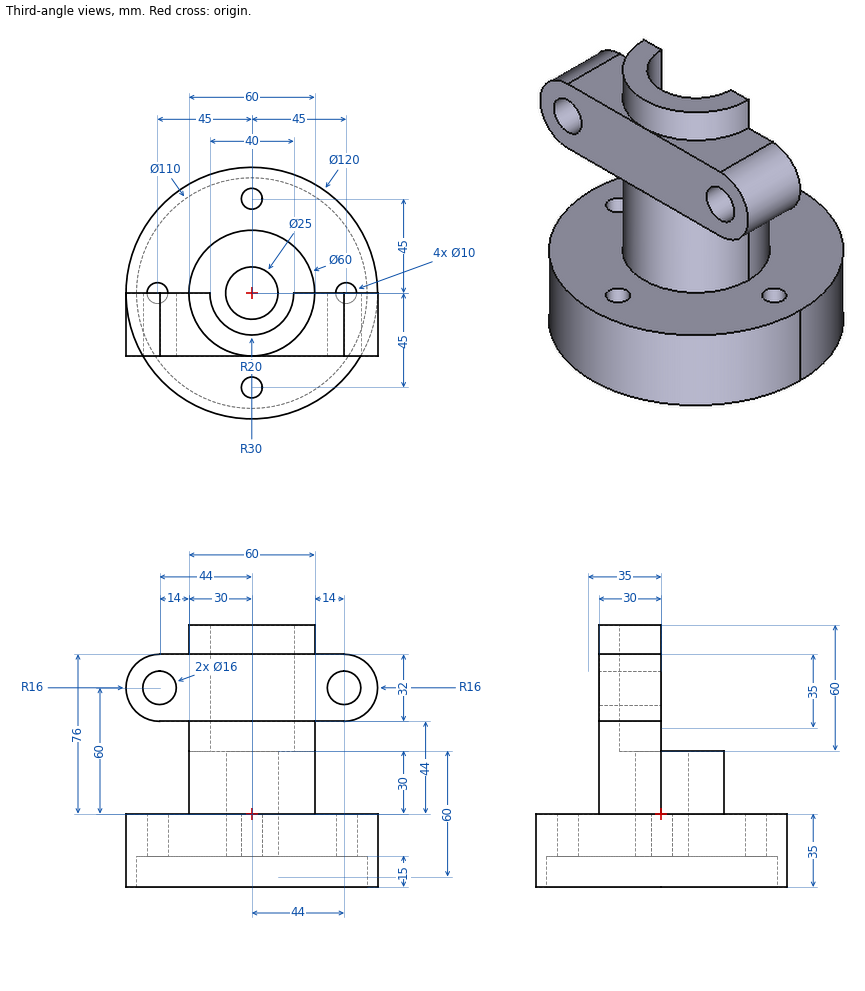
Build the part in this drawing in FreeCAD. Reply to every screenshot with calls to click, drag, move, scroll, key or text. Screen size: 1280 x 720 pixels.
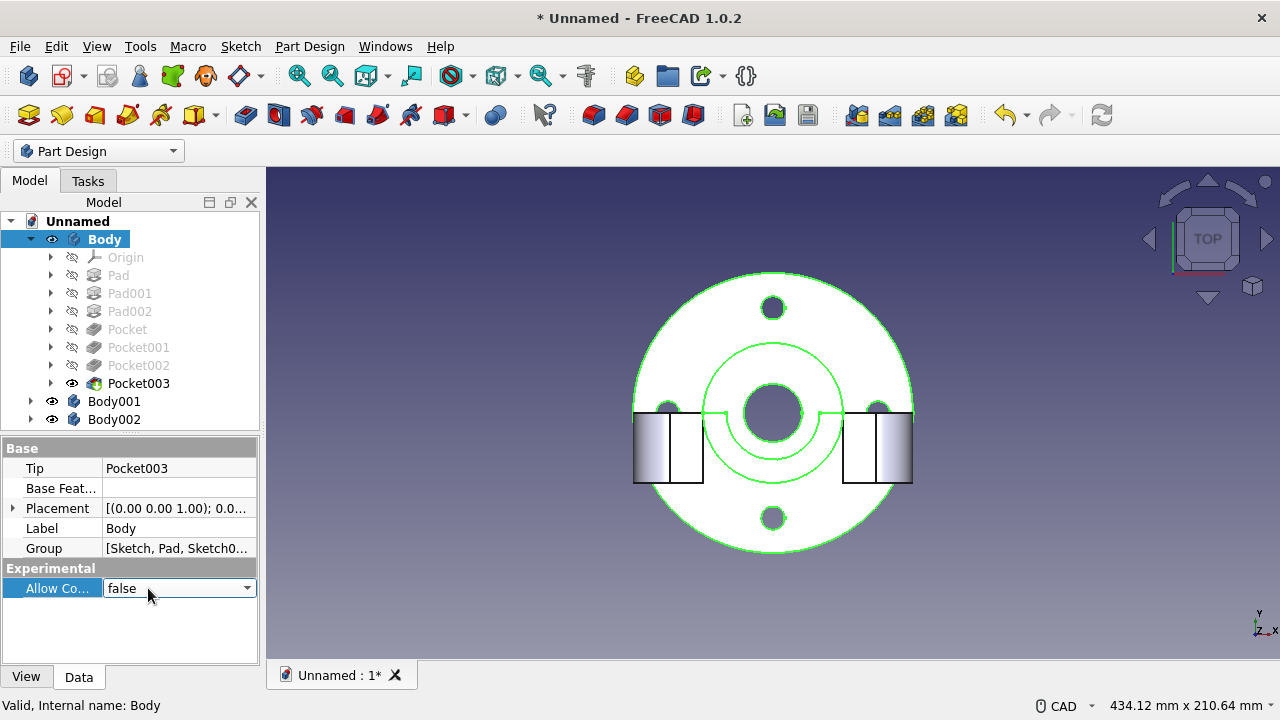
click(148, 588)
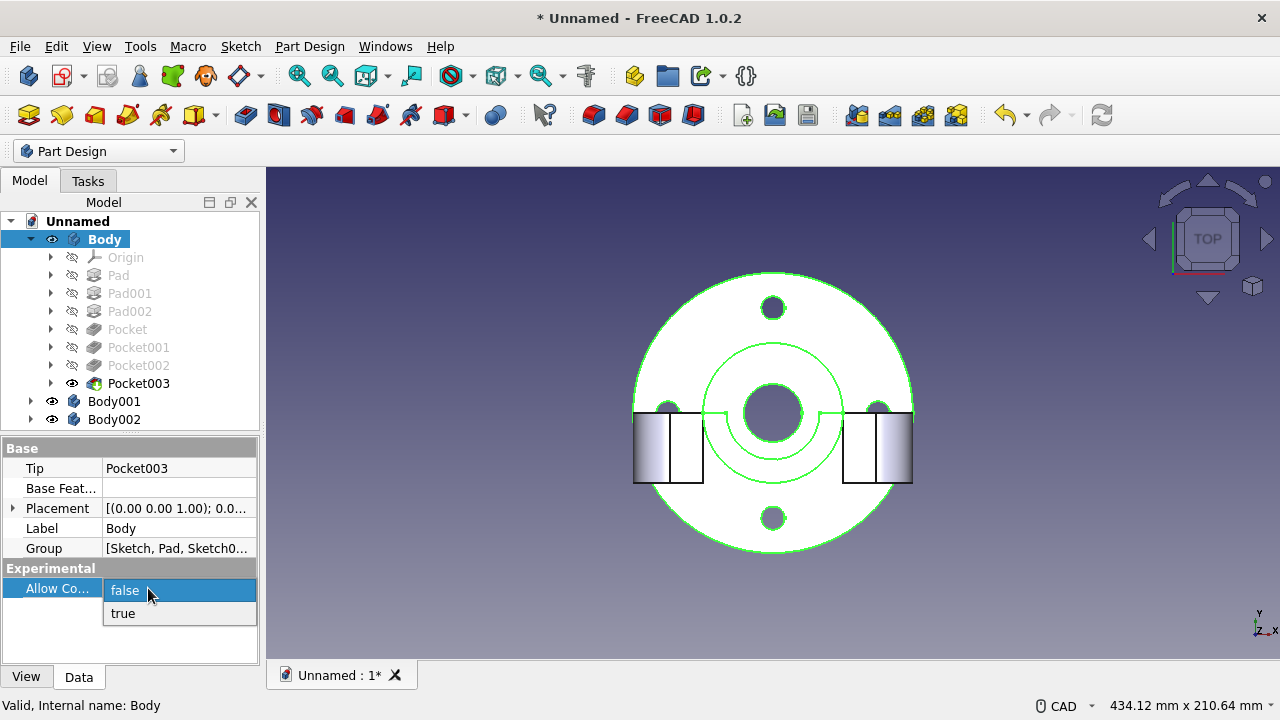
click(178, 614)
key(Return)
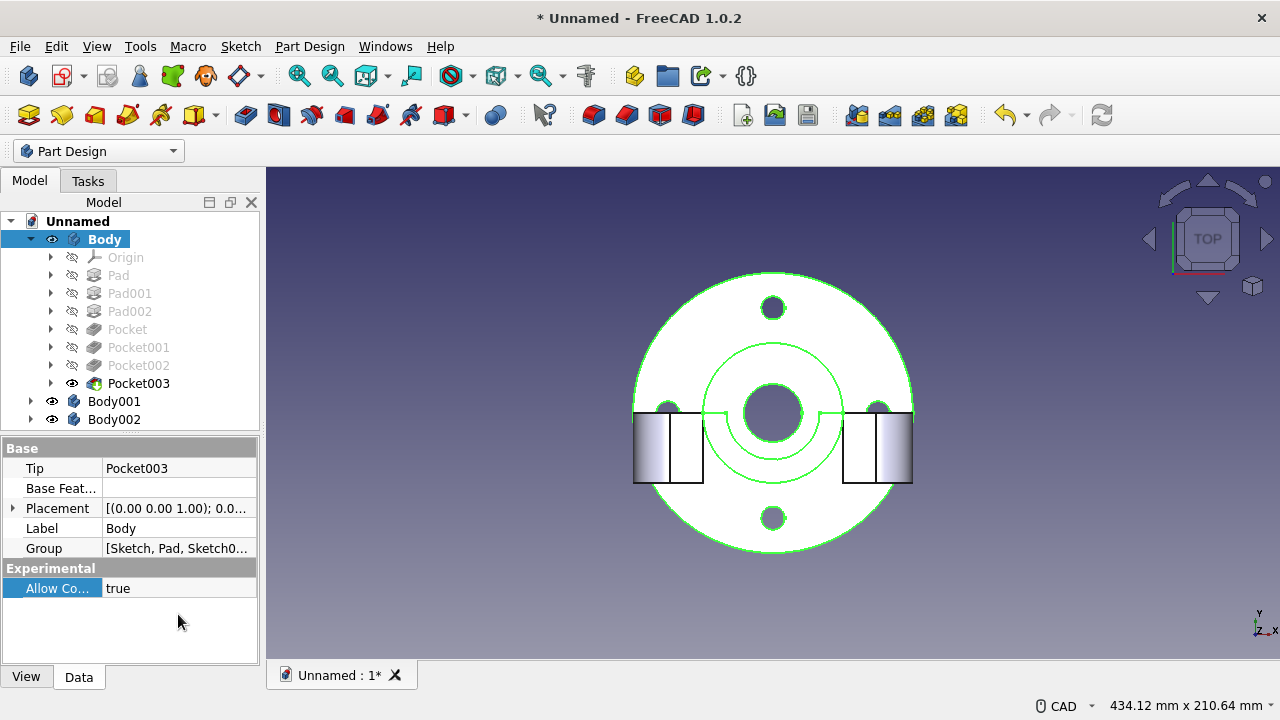
click(97, 401)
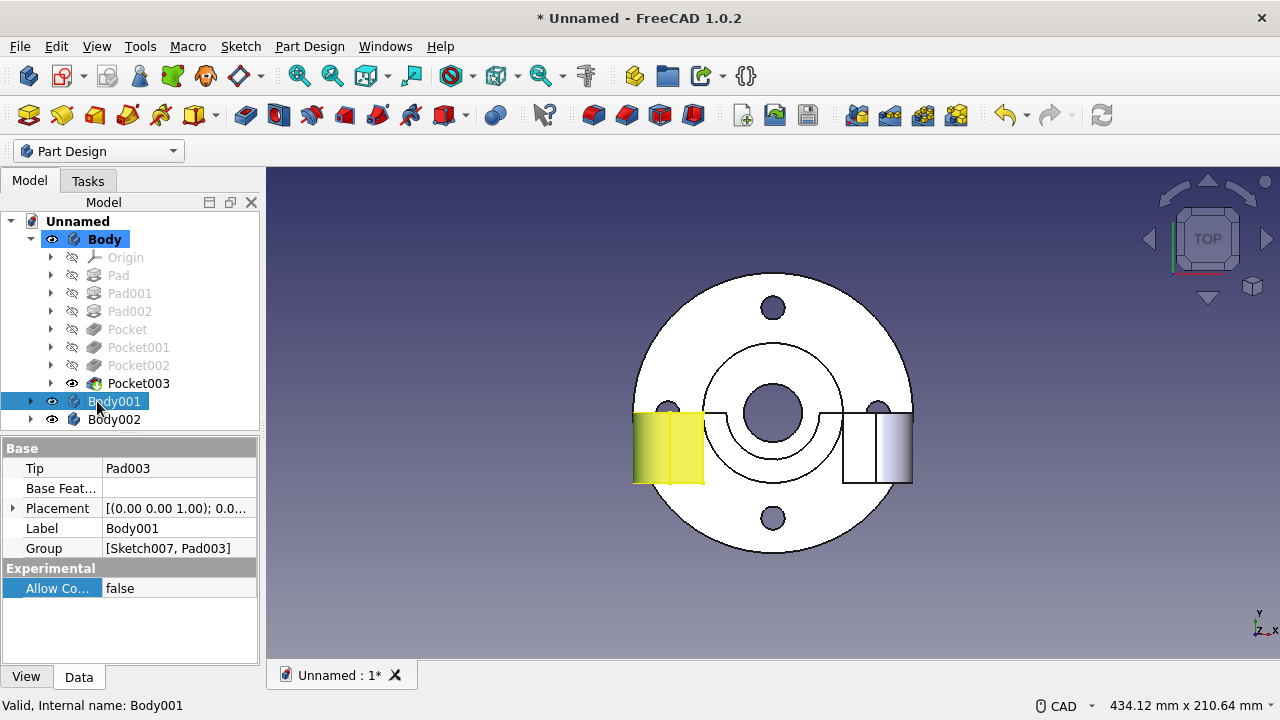
click(496, 116)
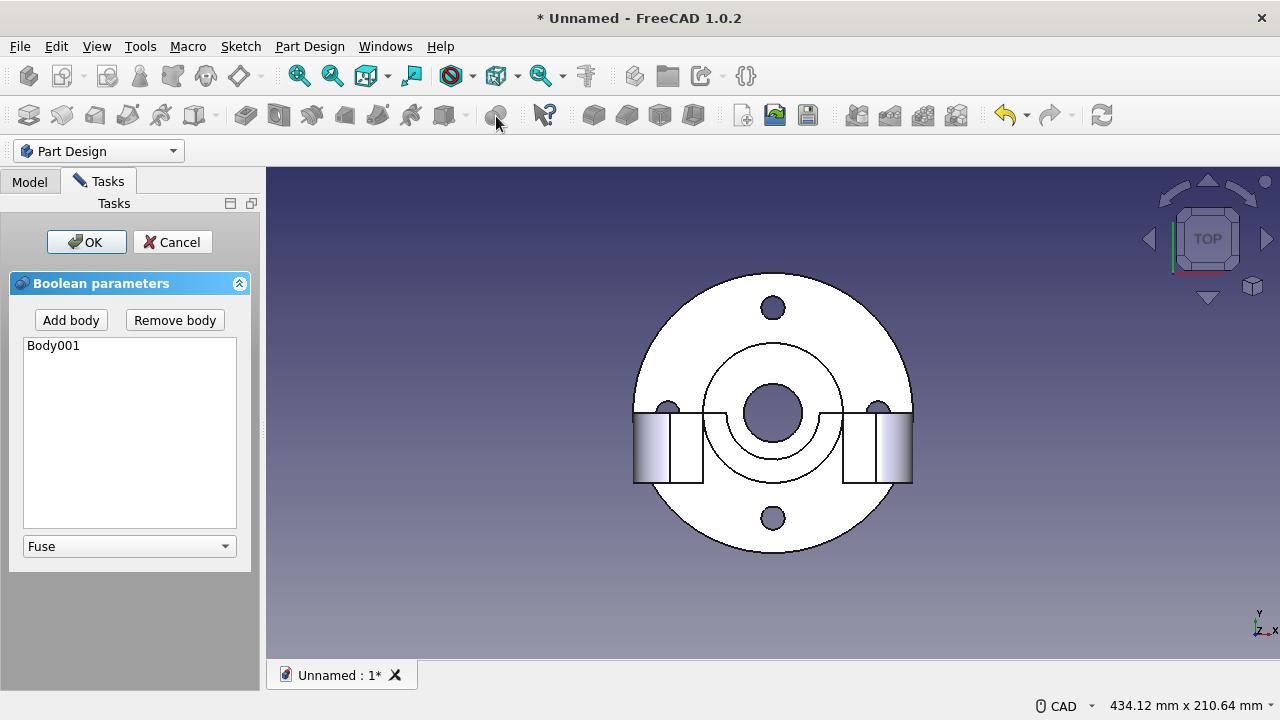
click(87, 242)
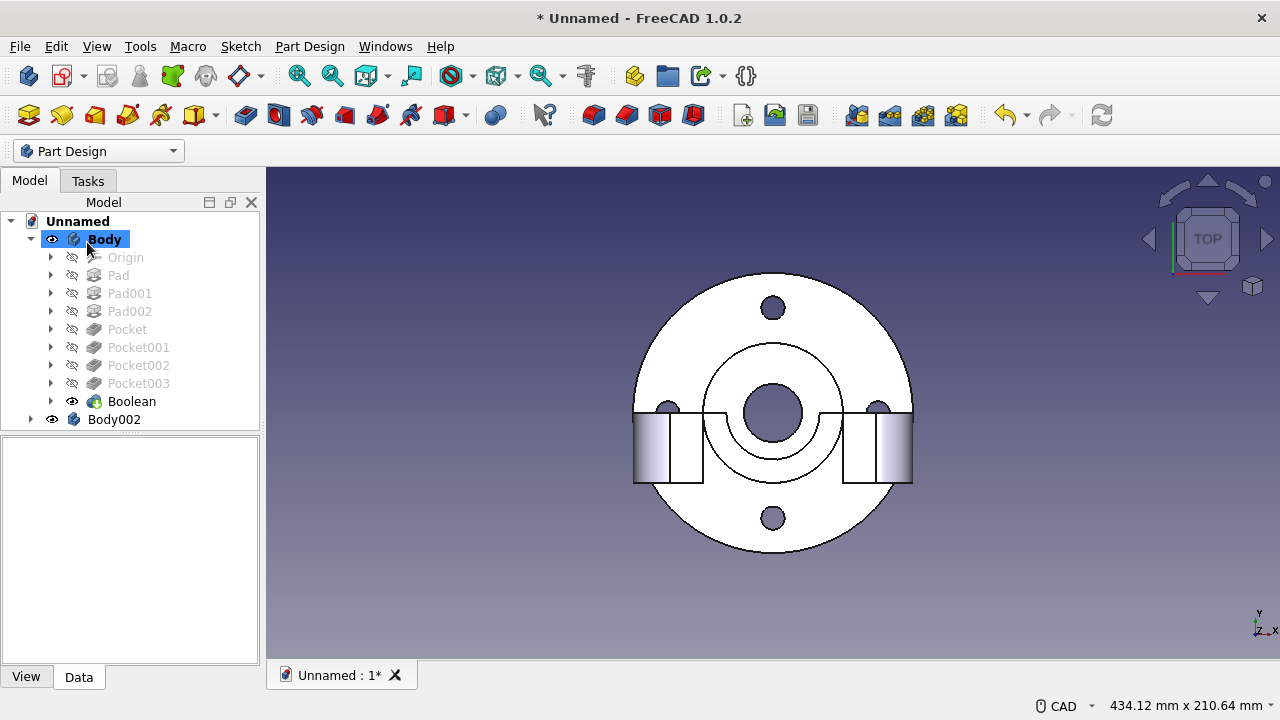
click(97, 419)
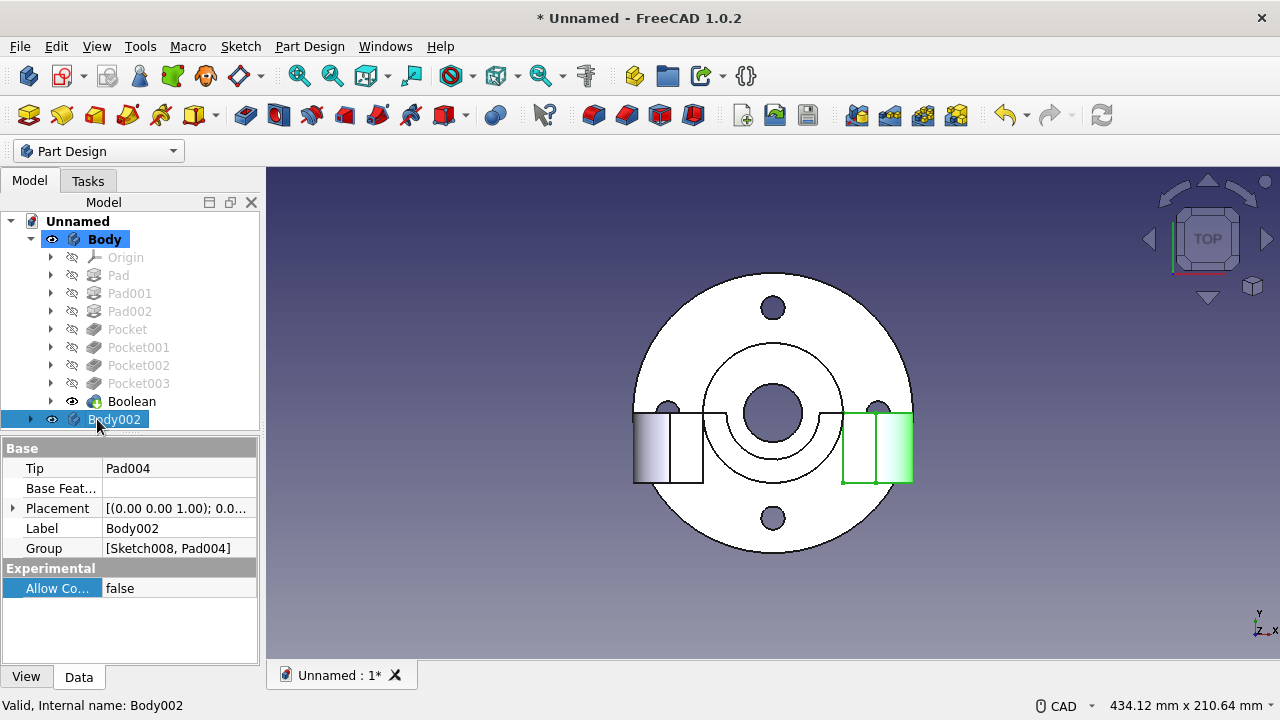
click(496, 116)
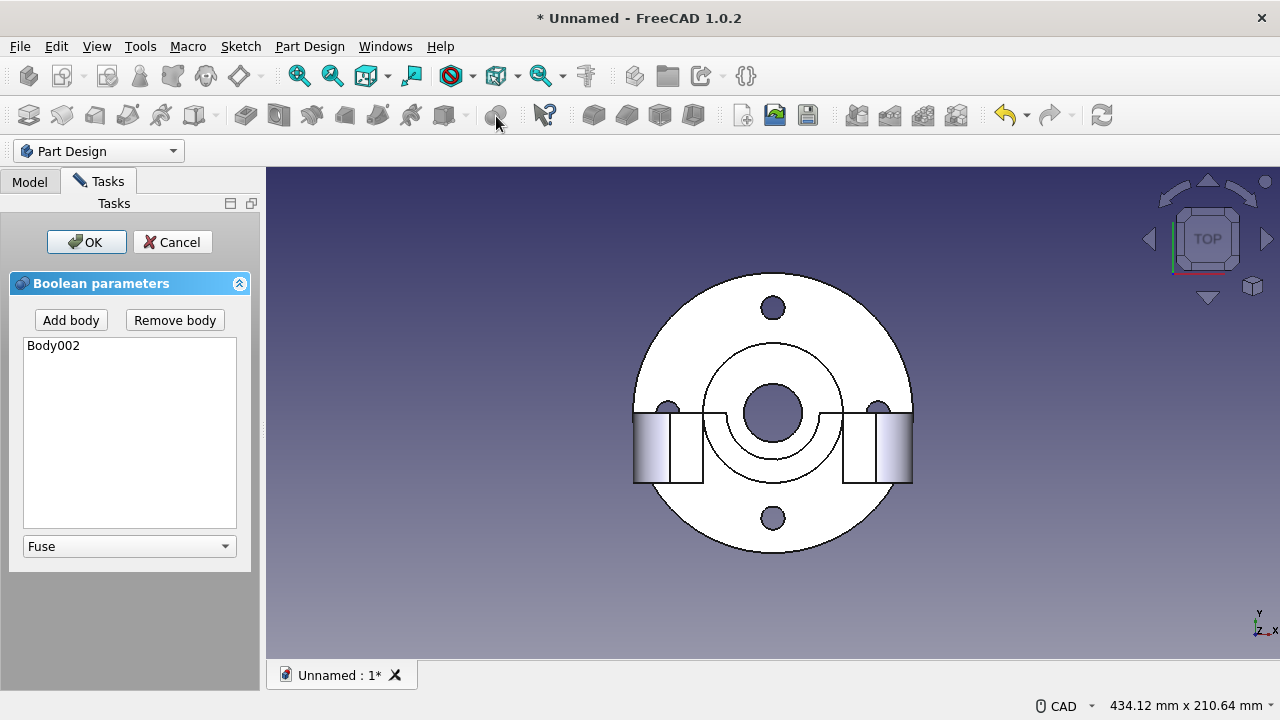
click(87, 242)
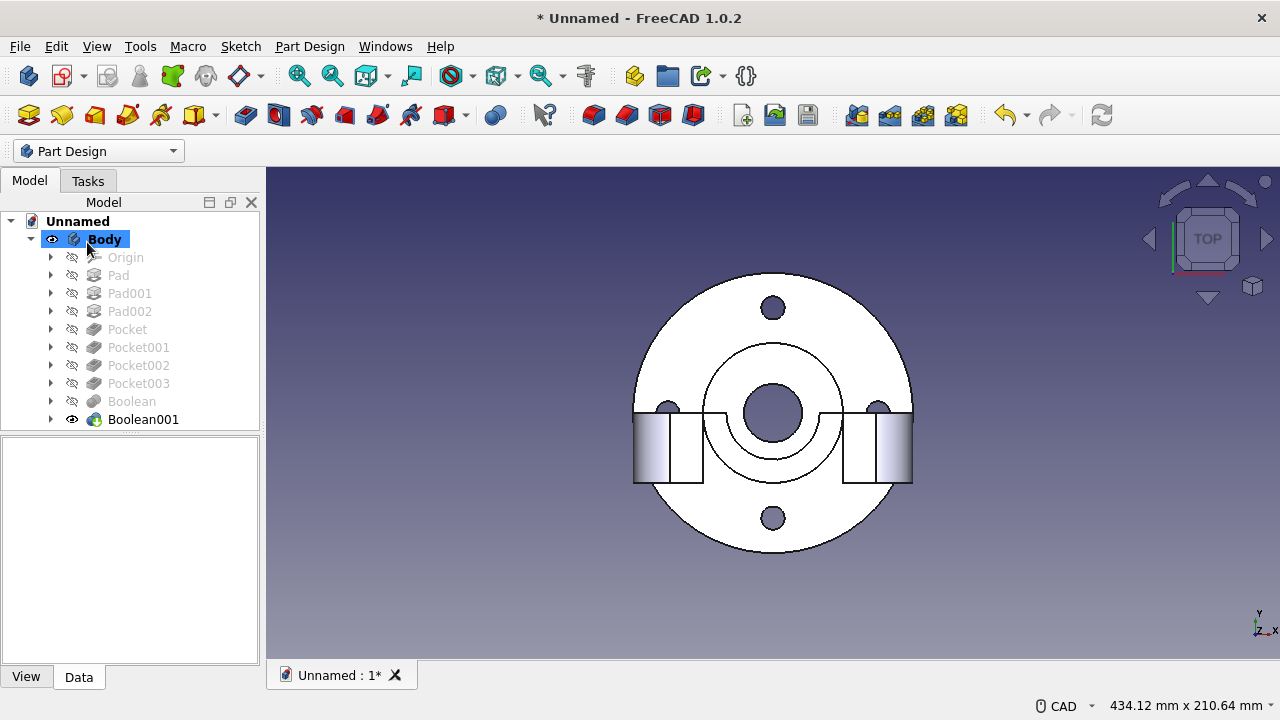
key(0)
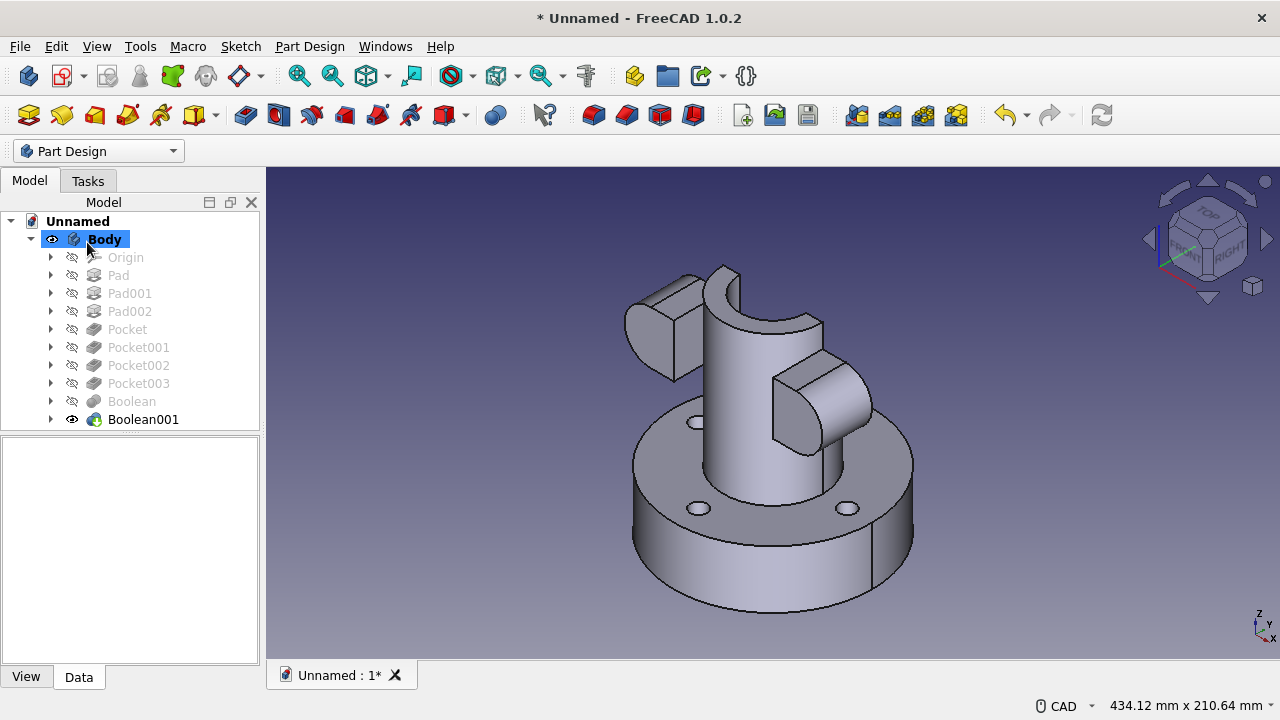
click(649, 336)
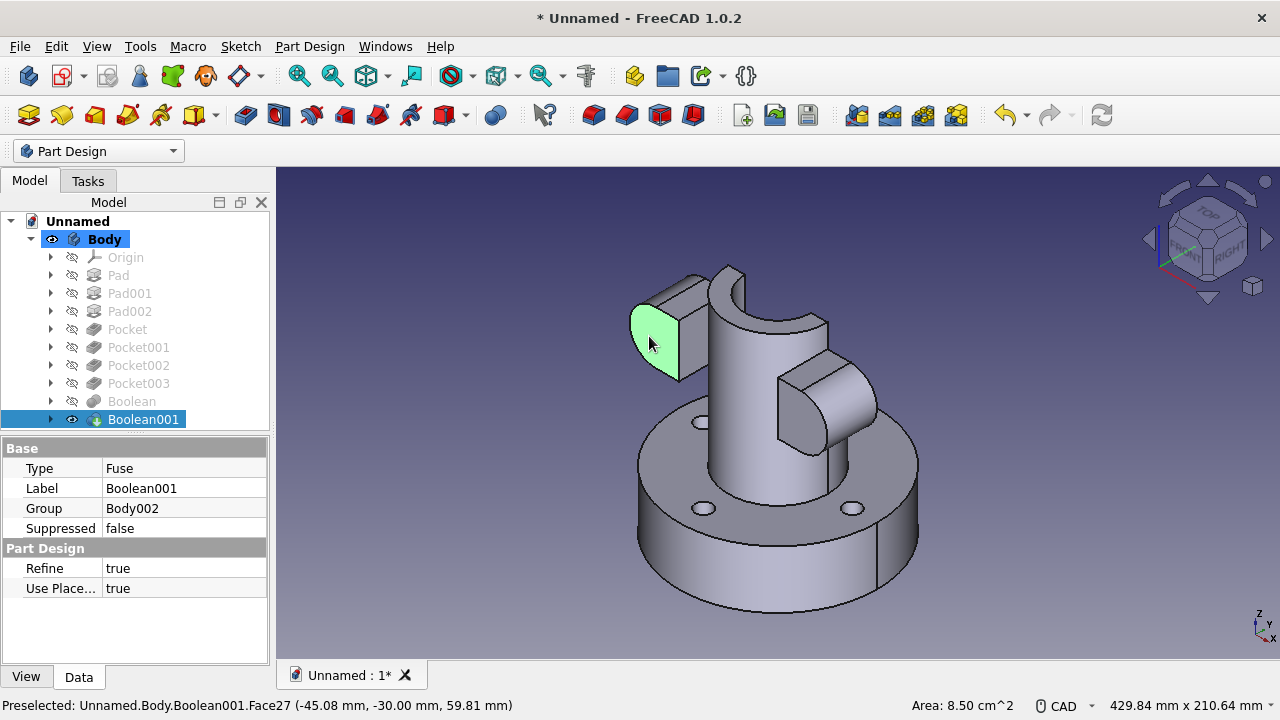
click(62, 76)